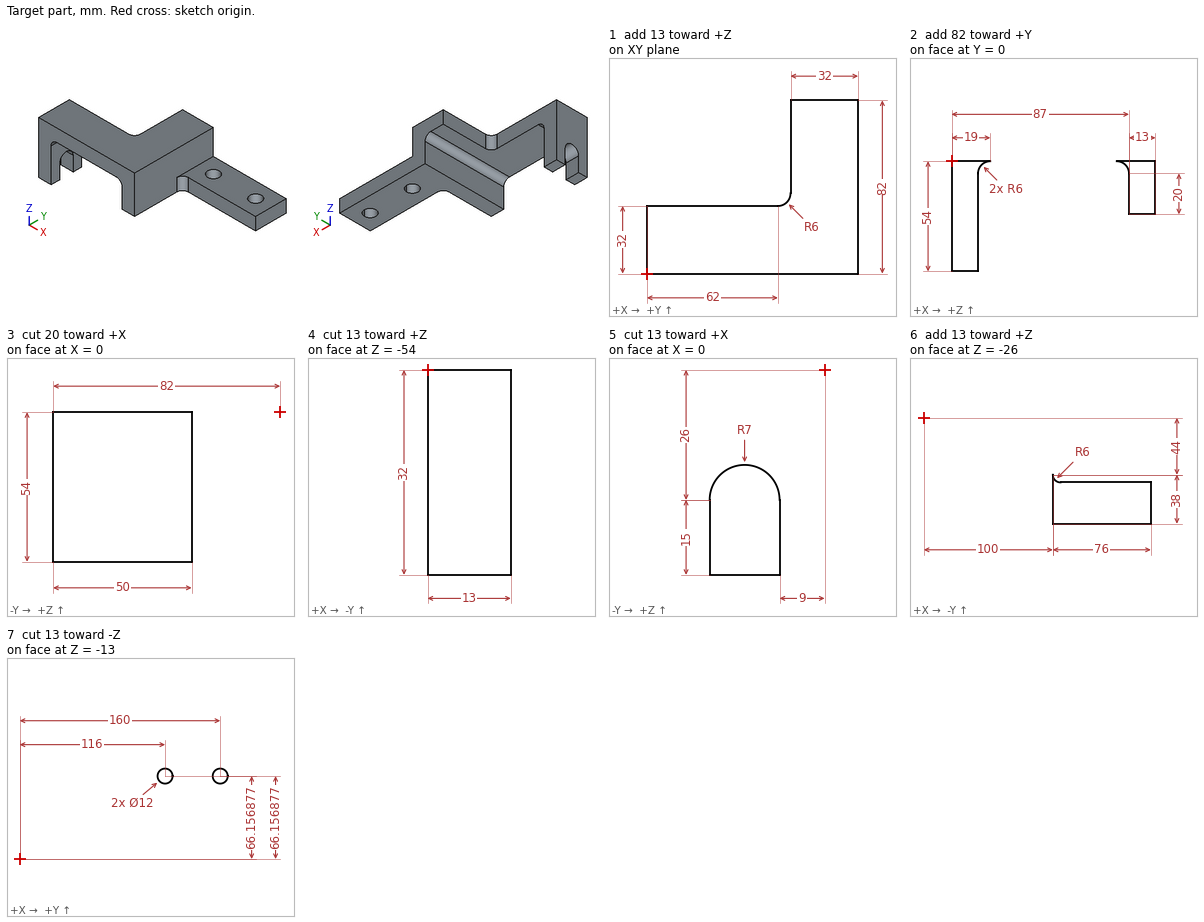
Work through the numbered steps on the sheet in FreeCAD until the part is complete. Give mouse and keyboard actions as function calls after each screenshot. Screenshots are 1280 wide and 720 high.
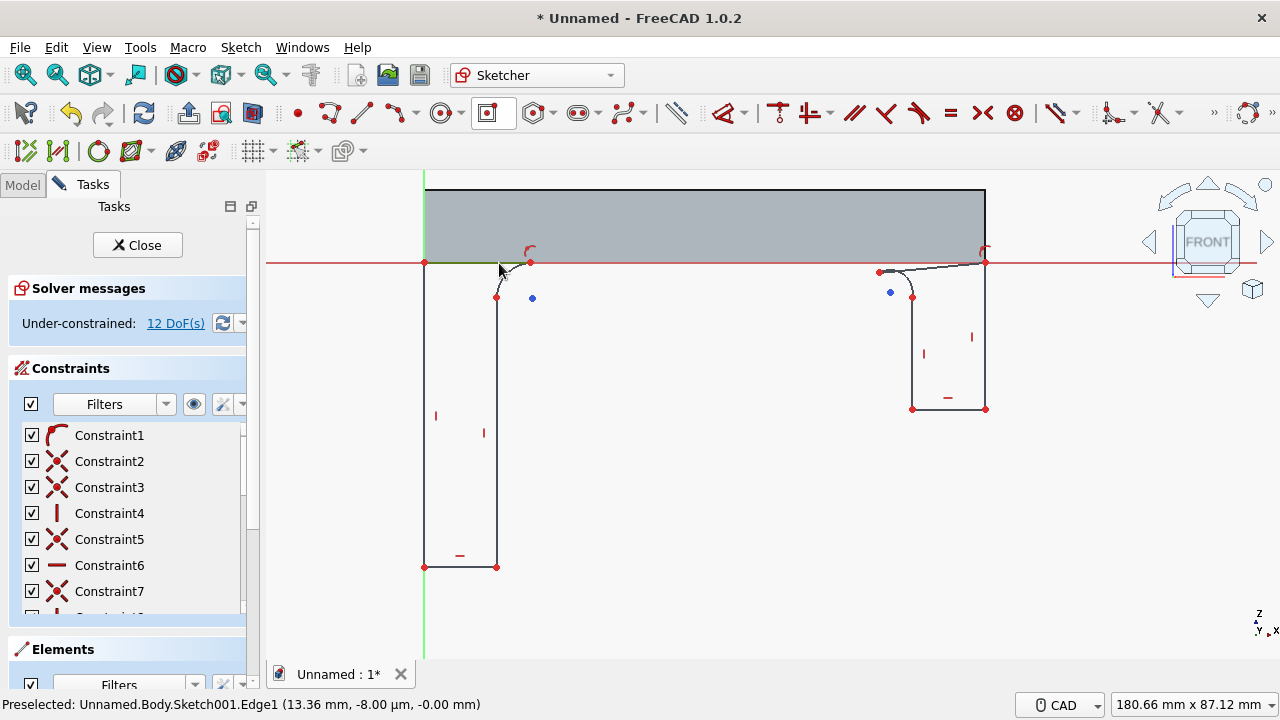
click(501, 282)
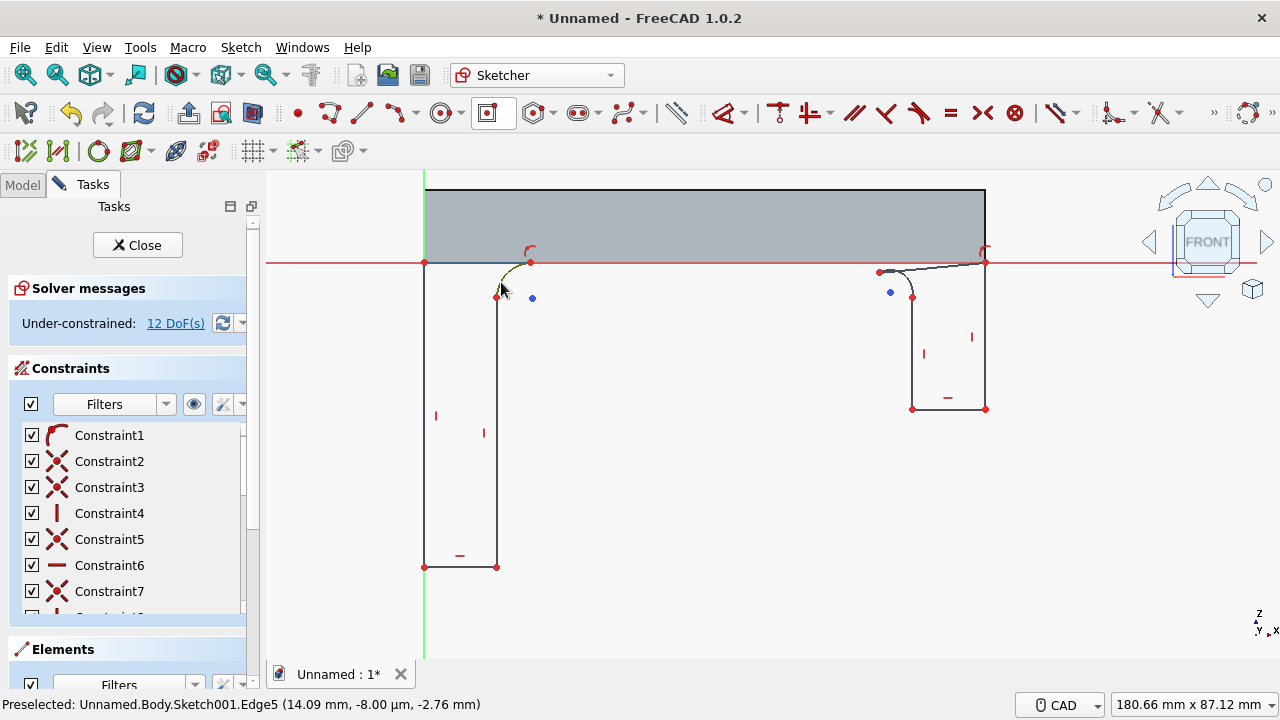
click(920, 114)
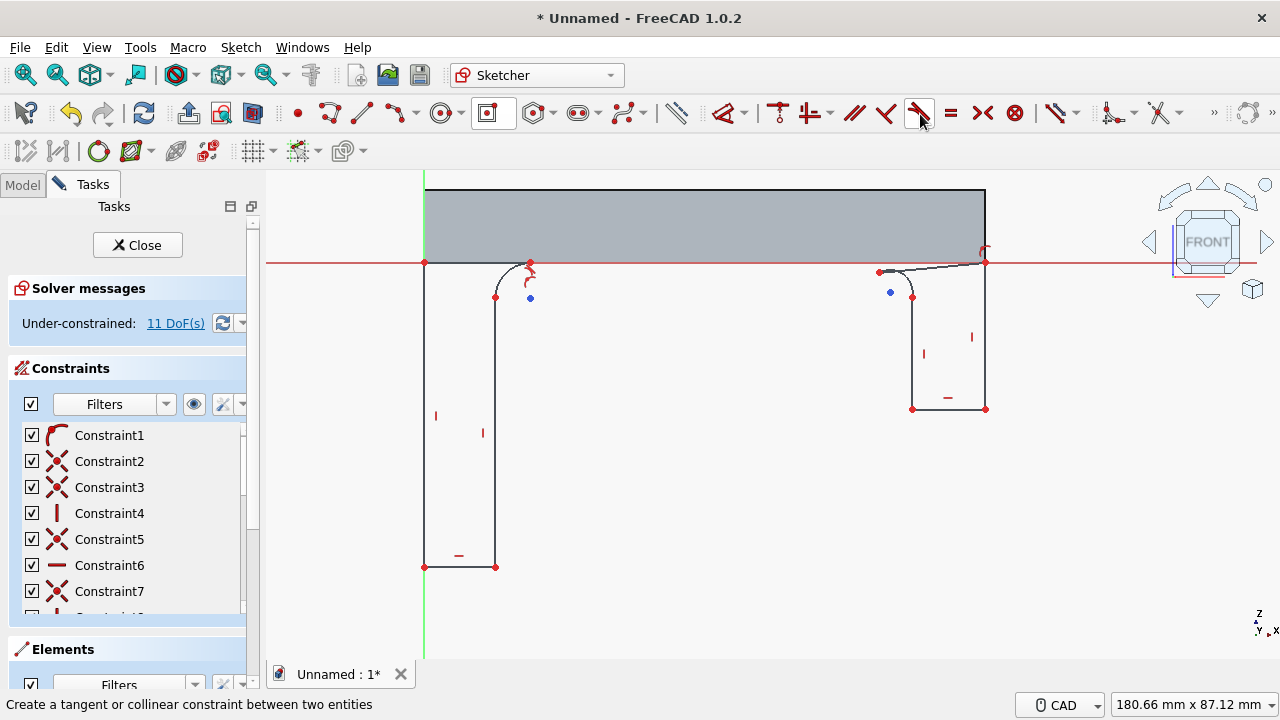
click(495, 486)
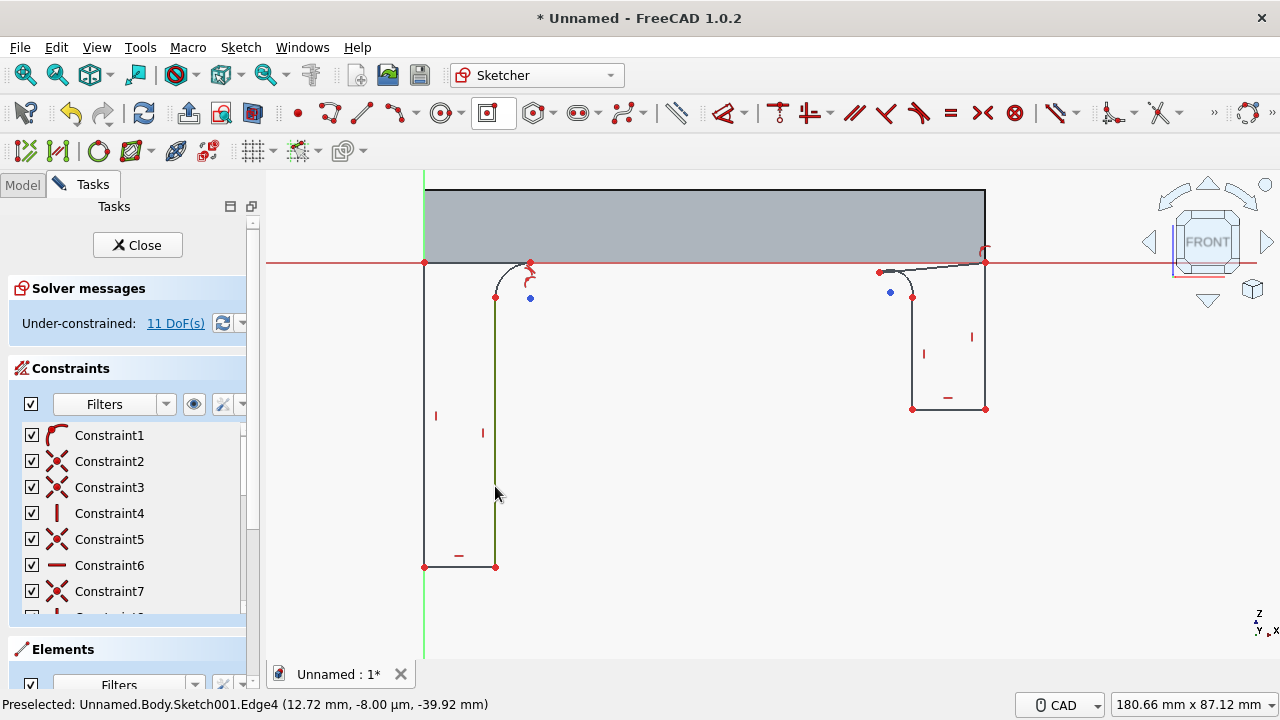
click(500, 282)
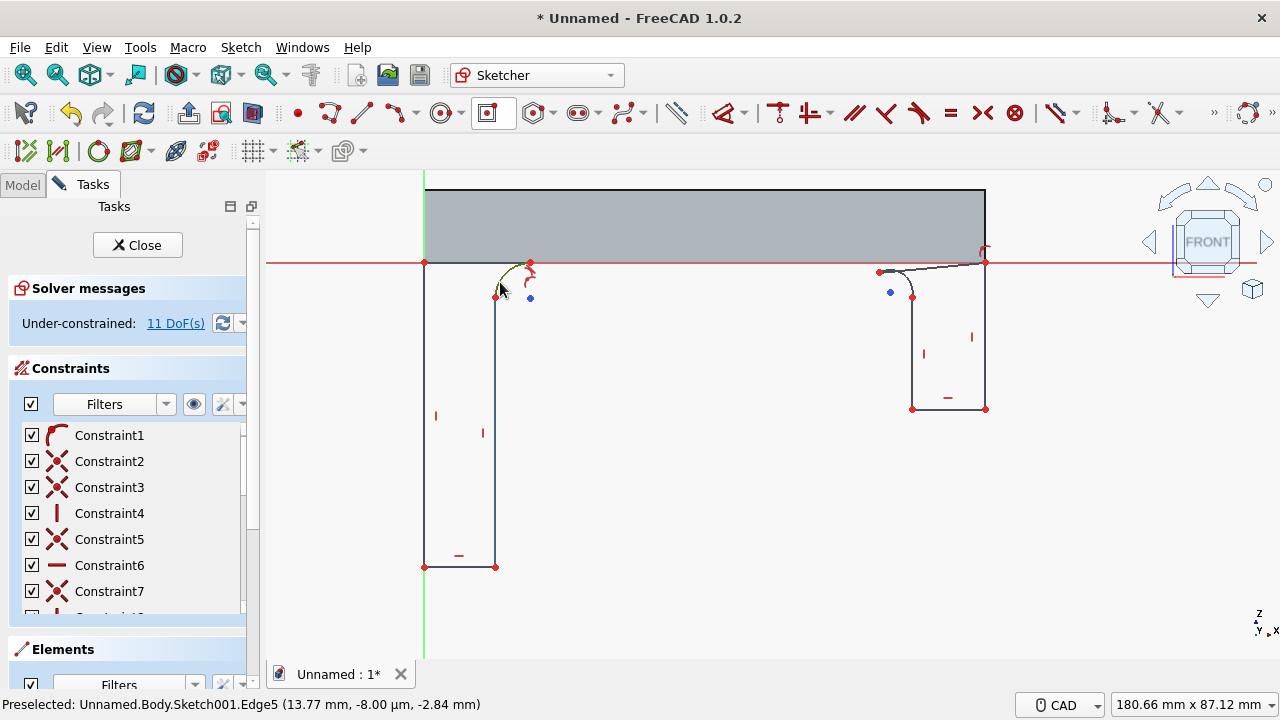
click(920, 114)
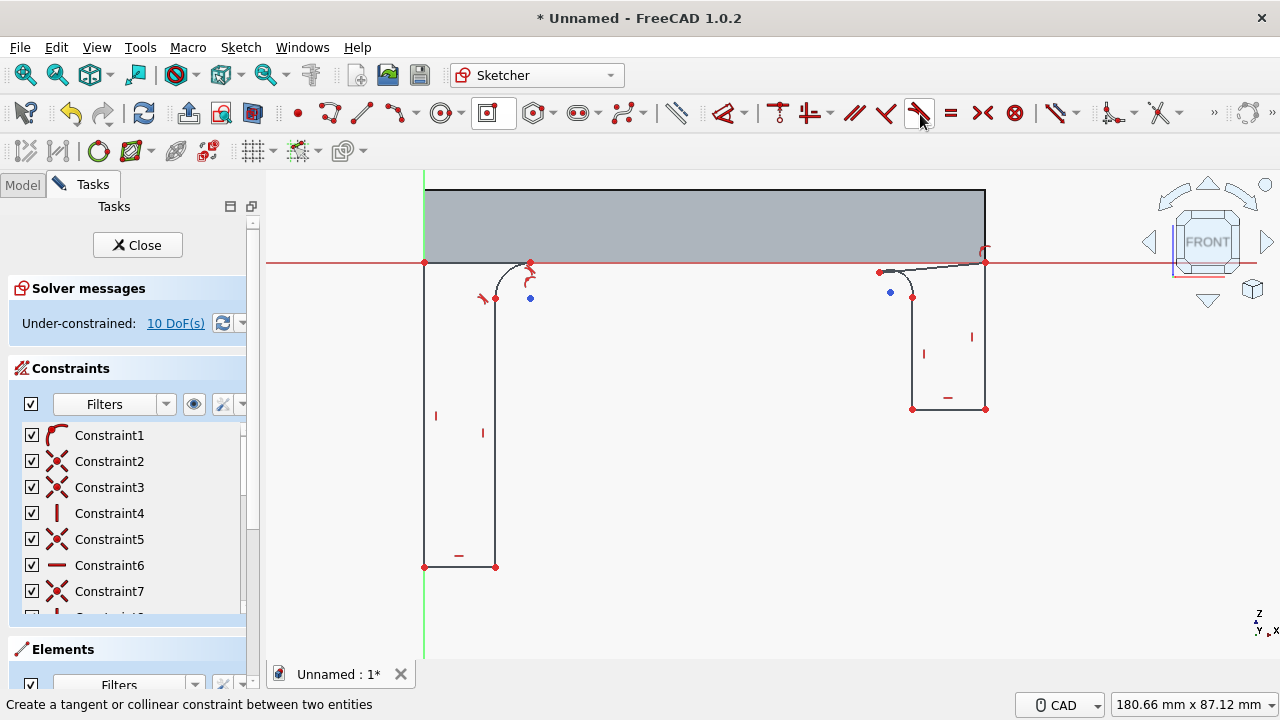
click(912, 332)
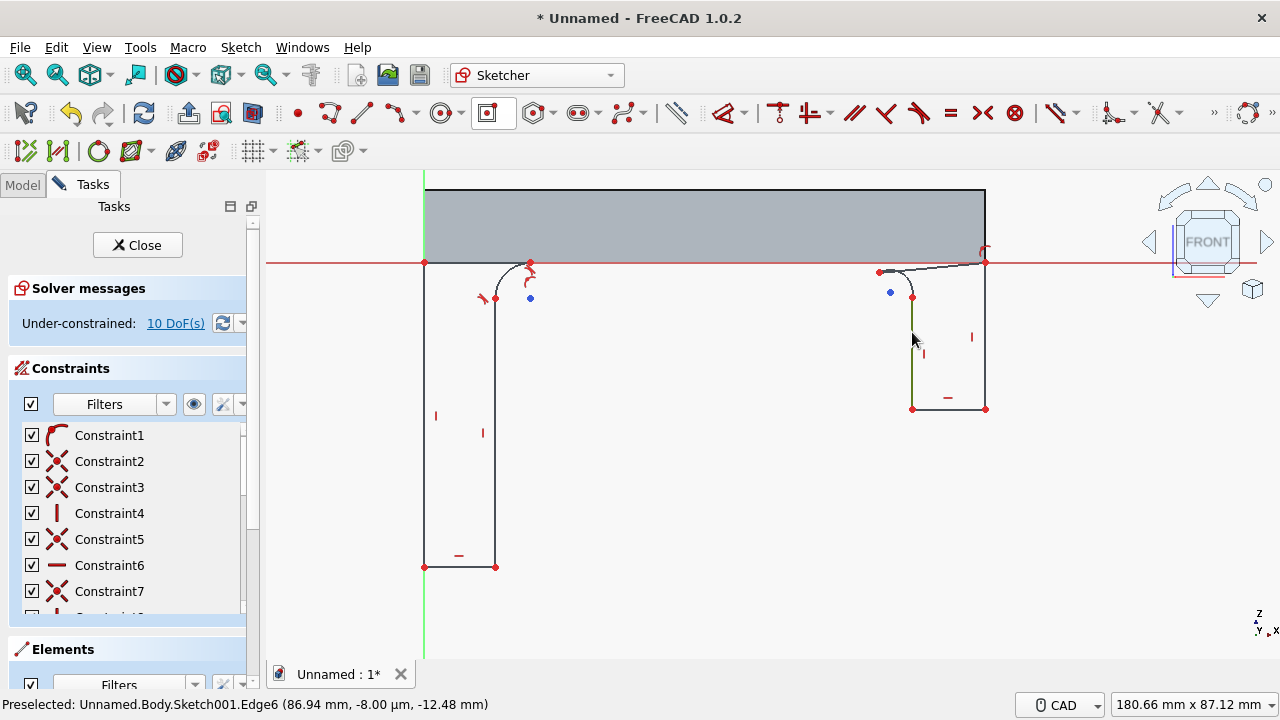
click(910, 283)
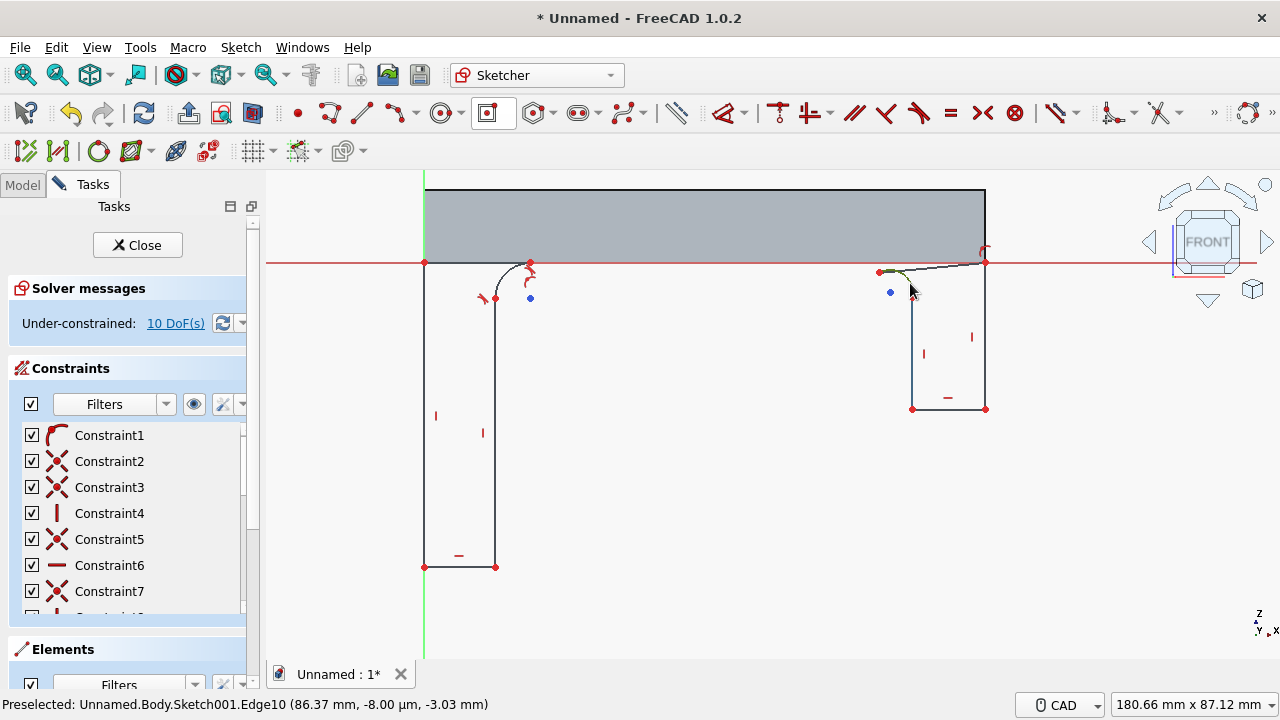
click(920, 114)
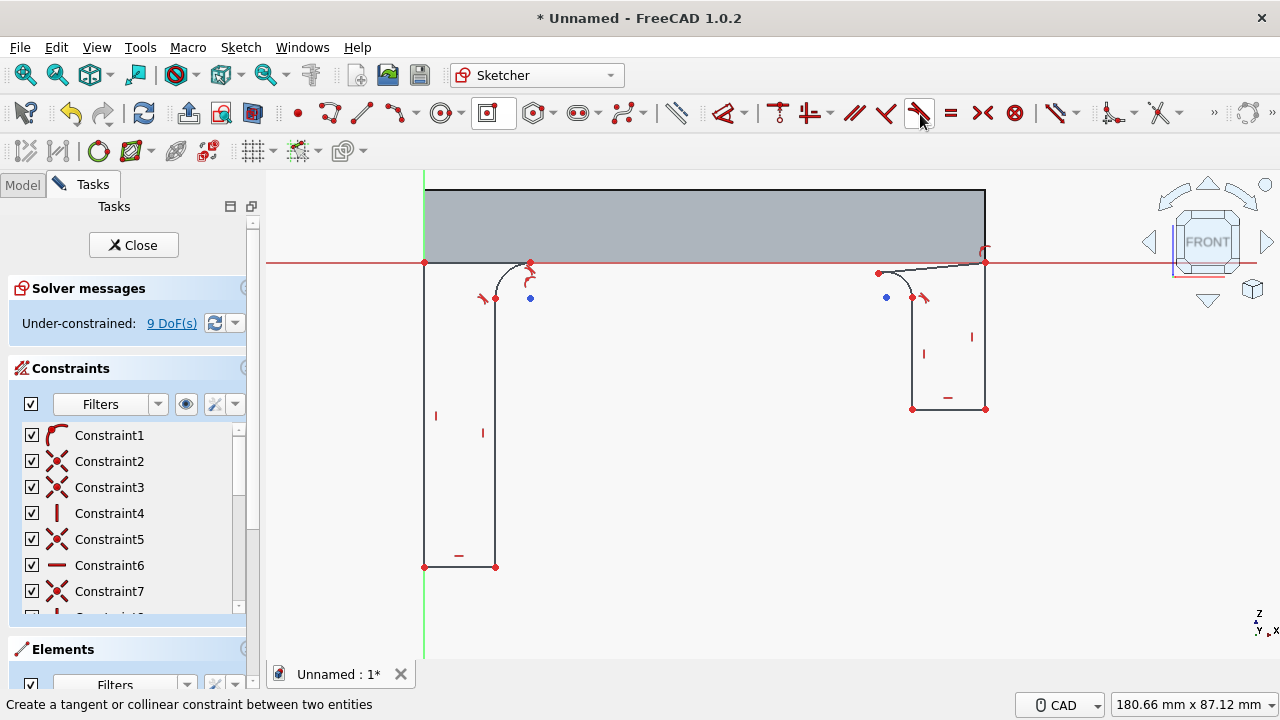
click(953, 266)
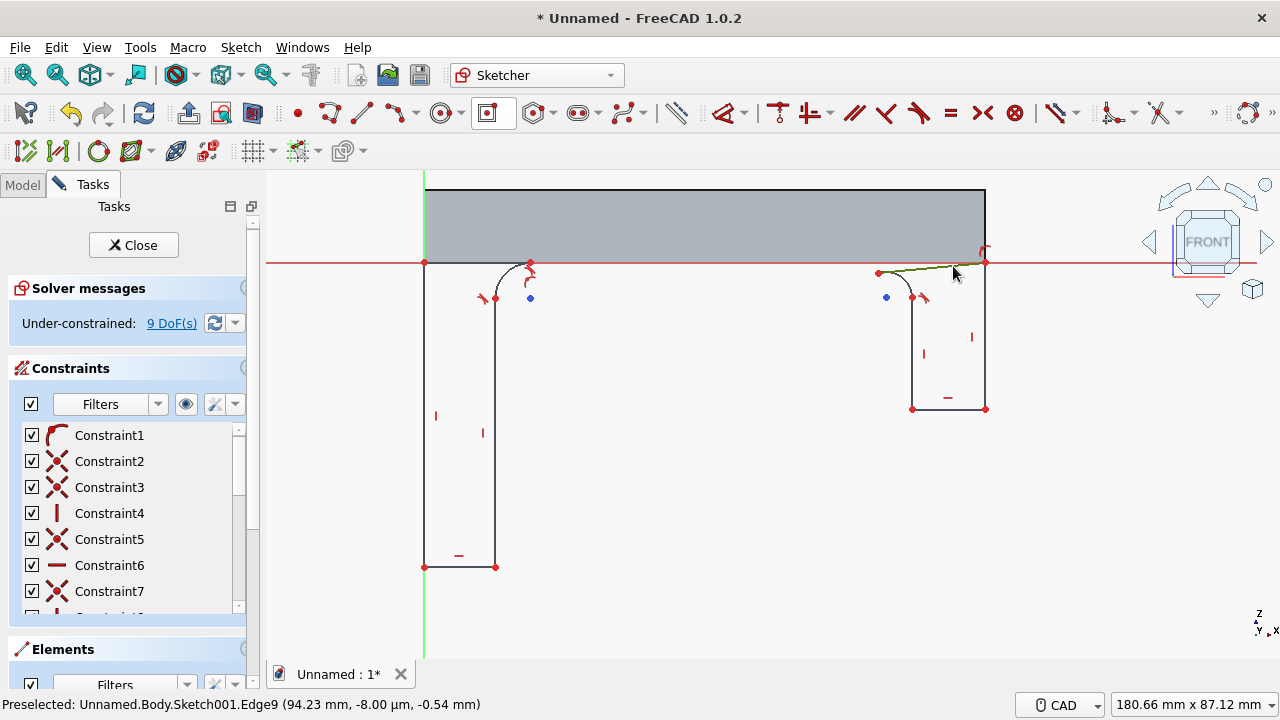
click(908, 284)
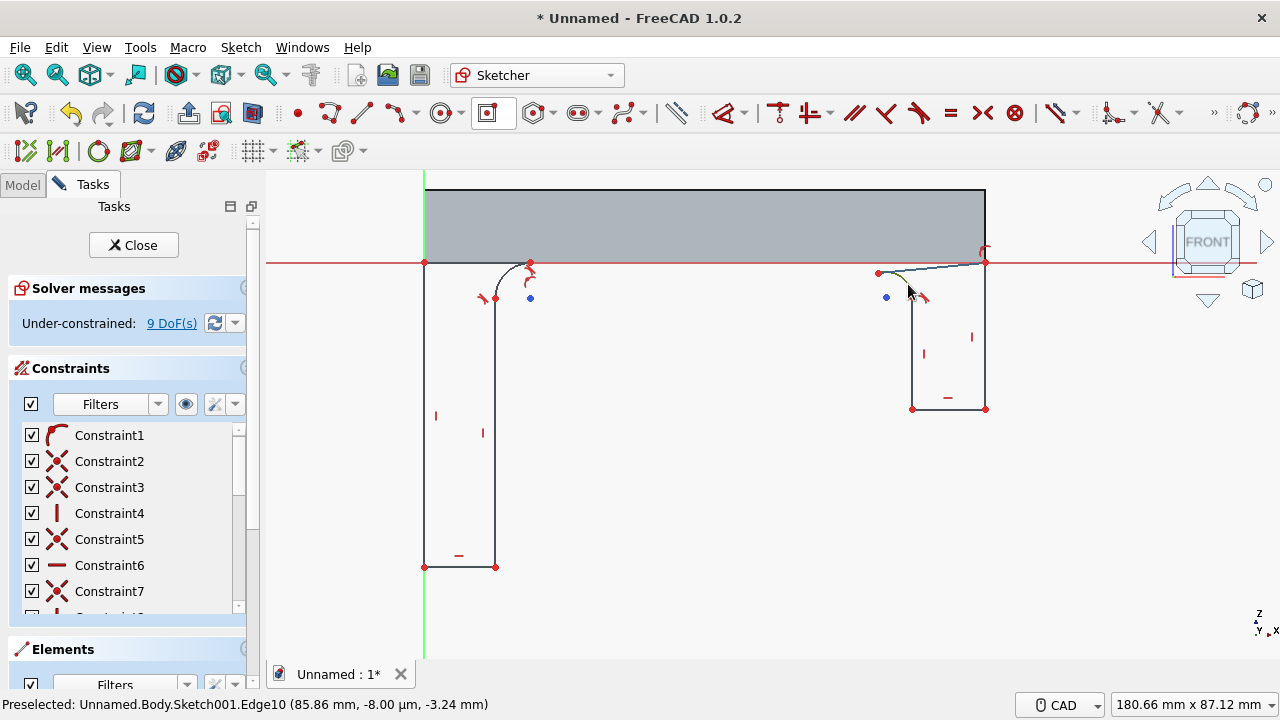
click(920, 114)